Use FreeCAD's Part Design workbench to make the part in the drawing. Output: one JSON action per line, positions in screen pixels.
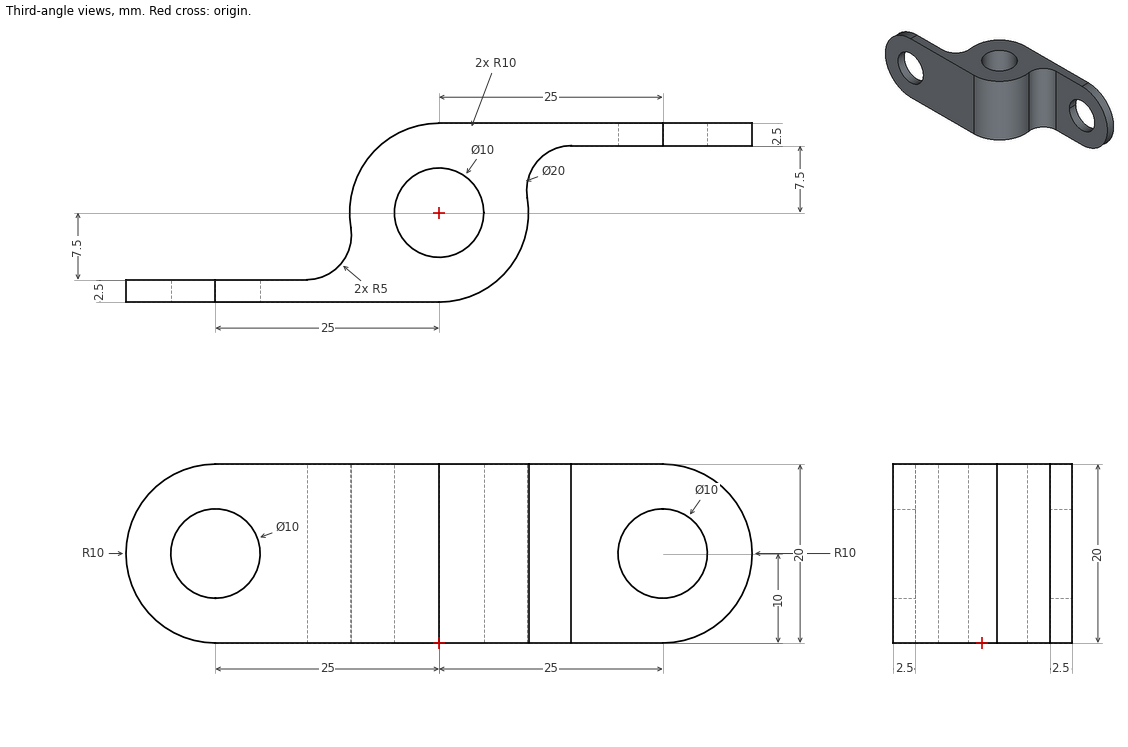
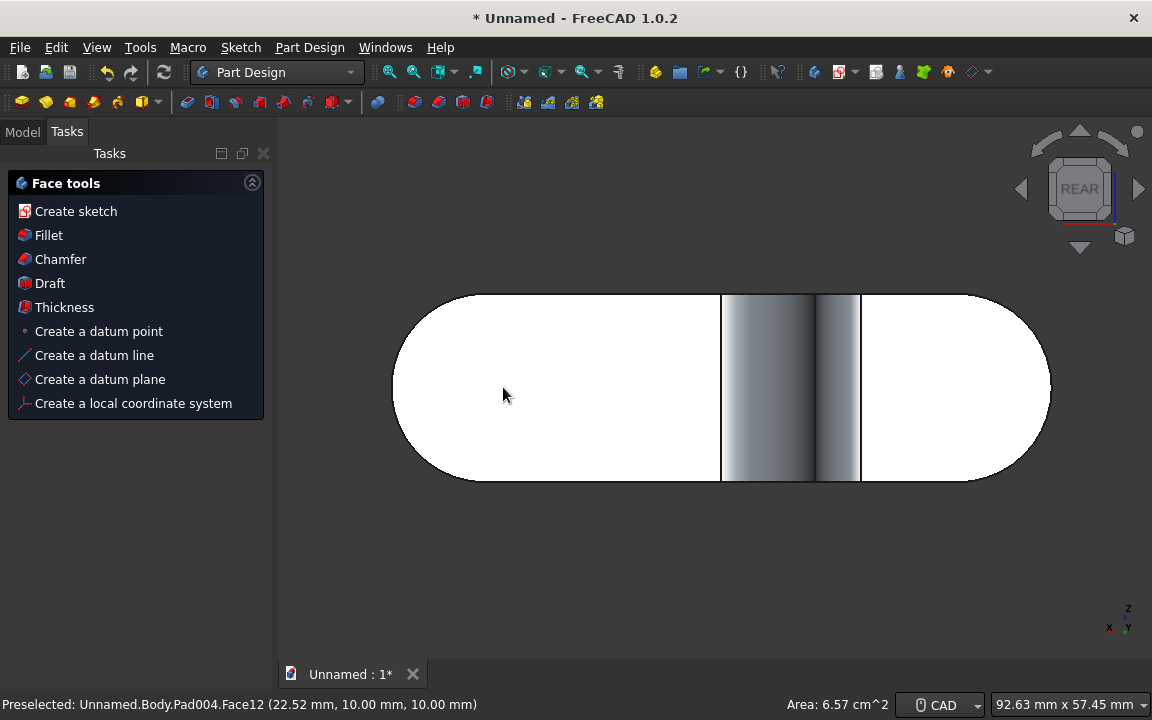
{"action": "left_click", "coordinate": [840, 72]}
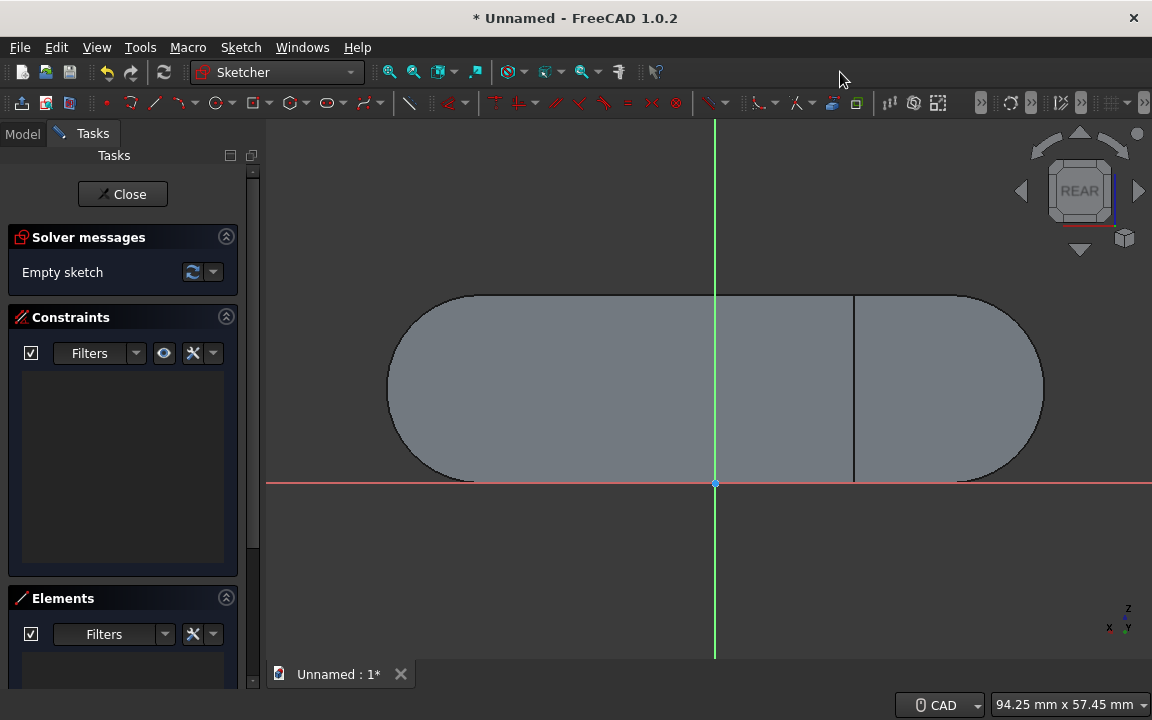
{"action": "scroll", "coordinate": [411, 389], "scroll_direction": "up", "scroll_amount": 6}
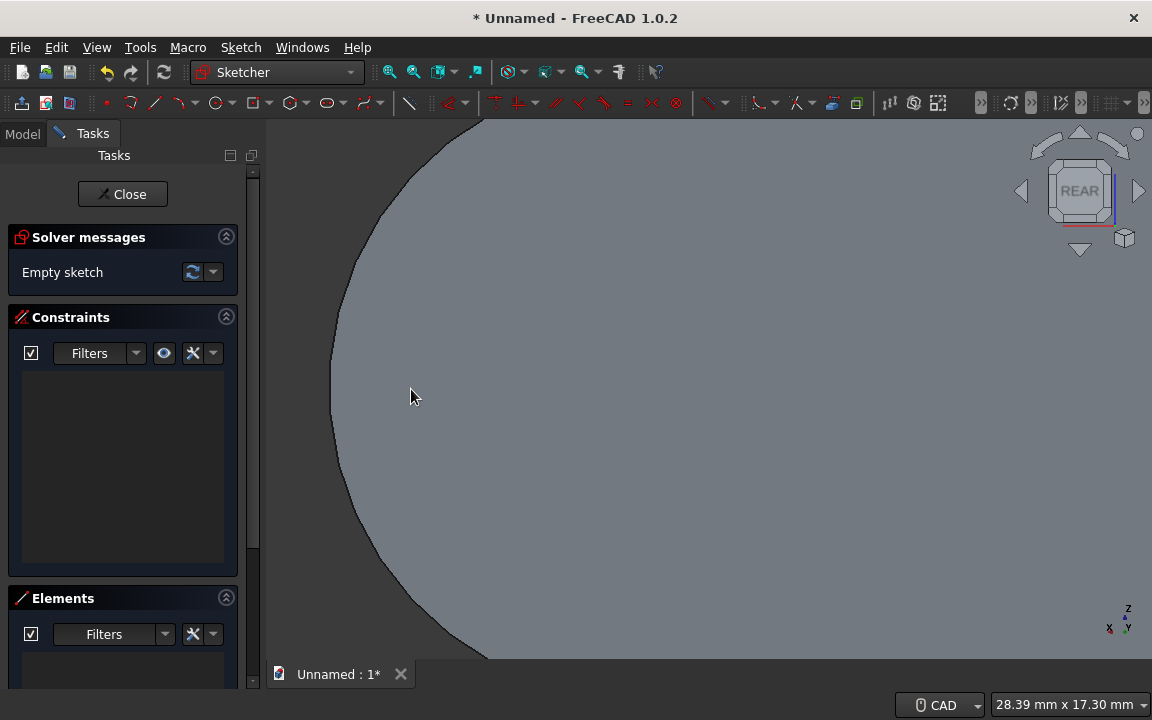
{"action": "key", "text": "g c"}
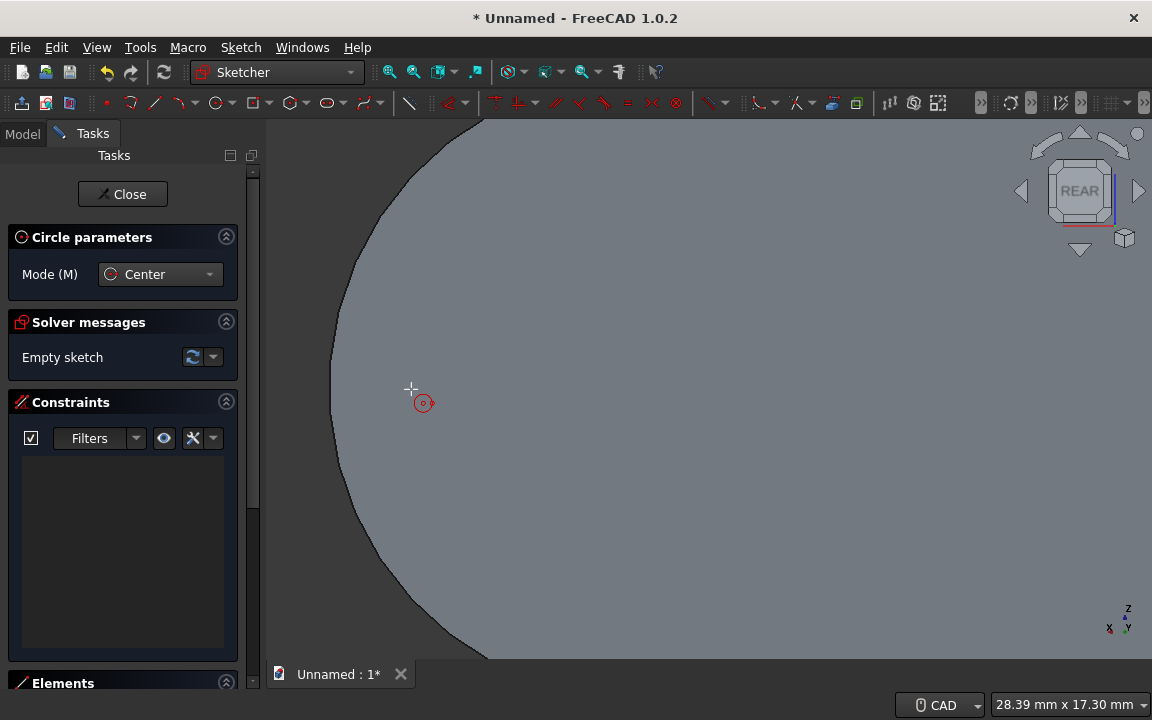
{"action": "left_click", "coordinate": [641, 388]}
{"action": "left_click", "coordinate": [752, 277]}
{"action": "key", "text": "Escape"}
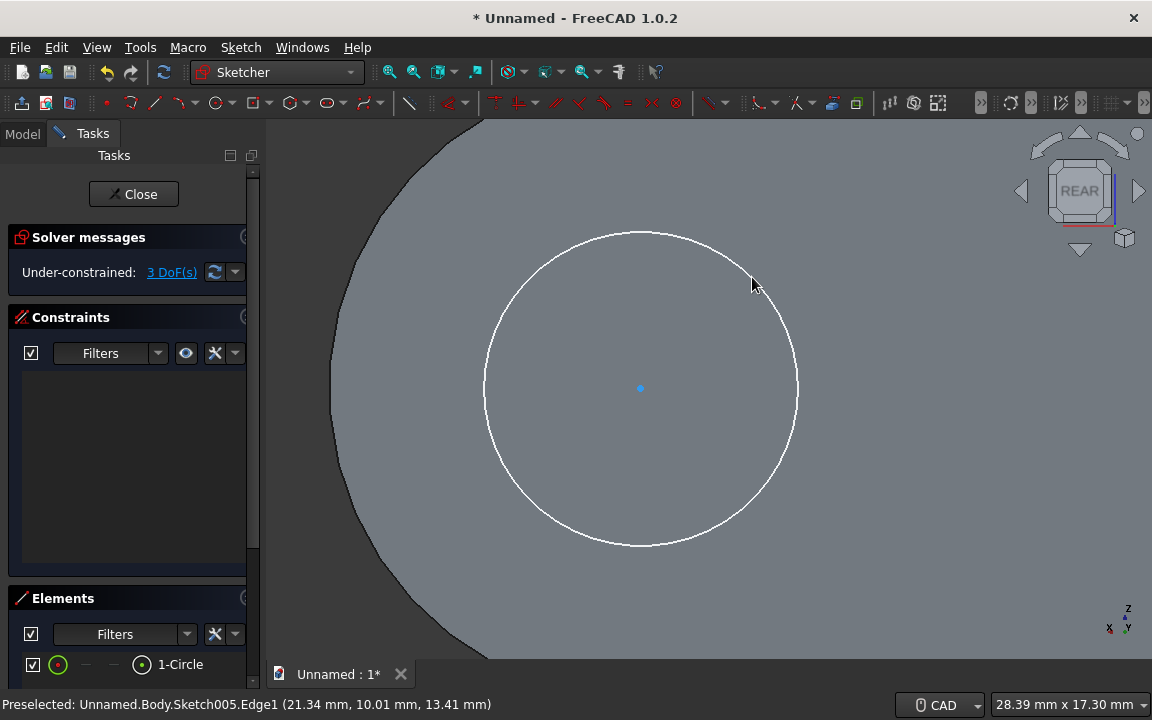
{"action": "key", "text": "d"}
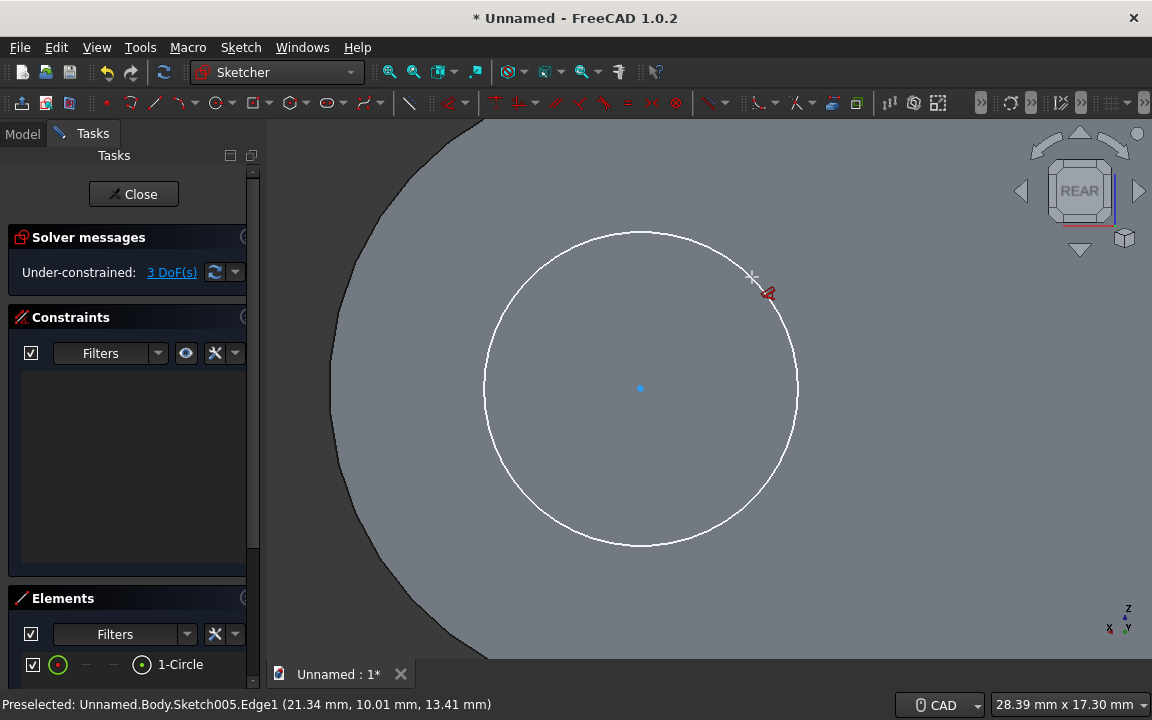
{"action": "left_click", "coordinate": [752, 278]}
{"action": "left_click", "coordinate": [775, 255]}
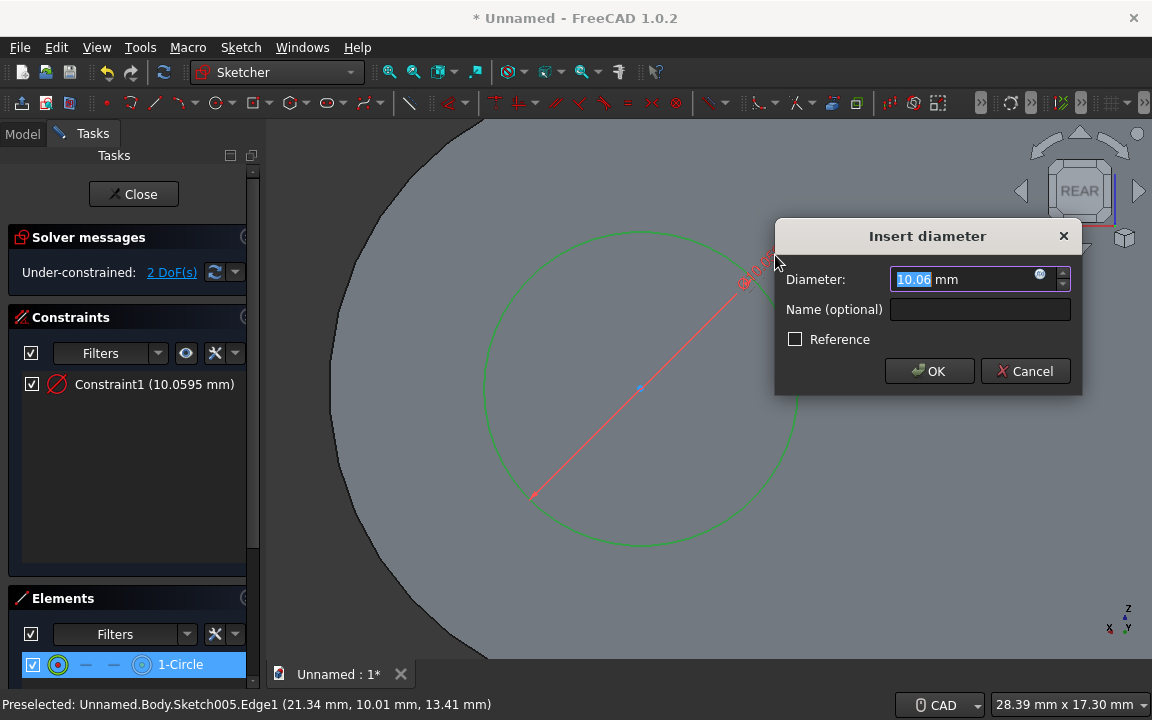
{"action": "type", "text": "10"}
{"action": "key", "text": "Return"}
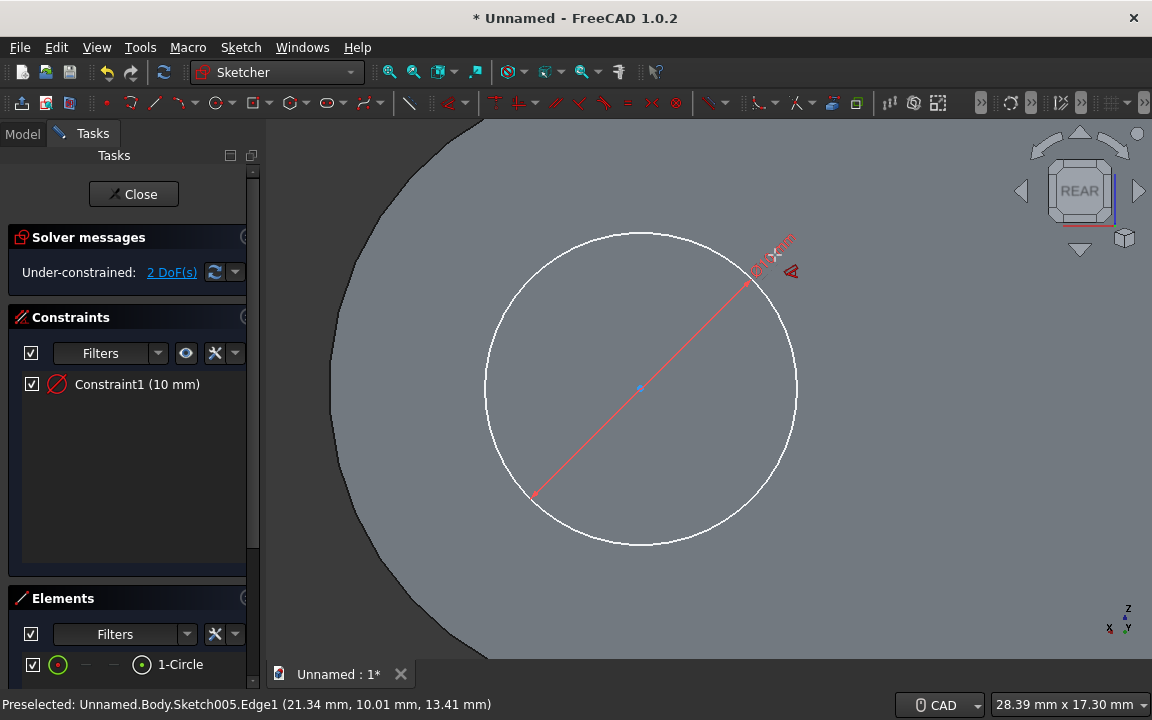
{"action": "left_click", "coordinate": [641, 389]}
{"action": "left_click", "coordinate": [814, 355]}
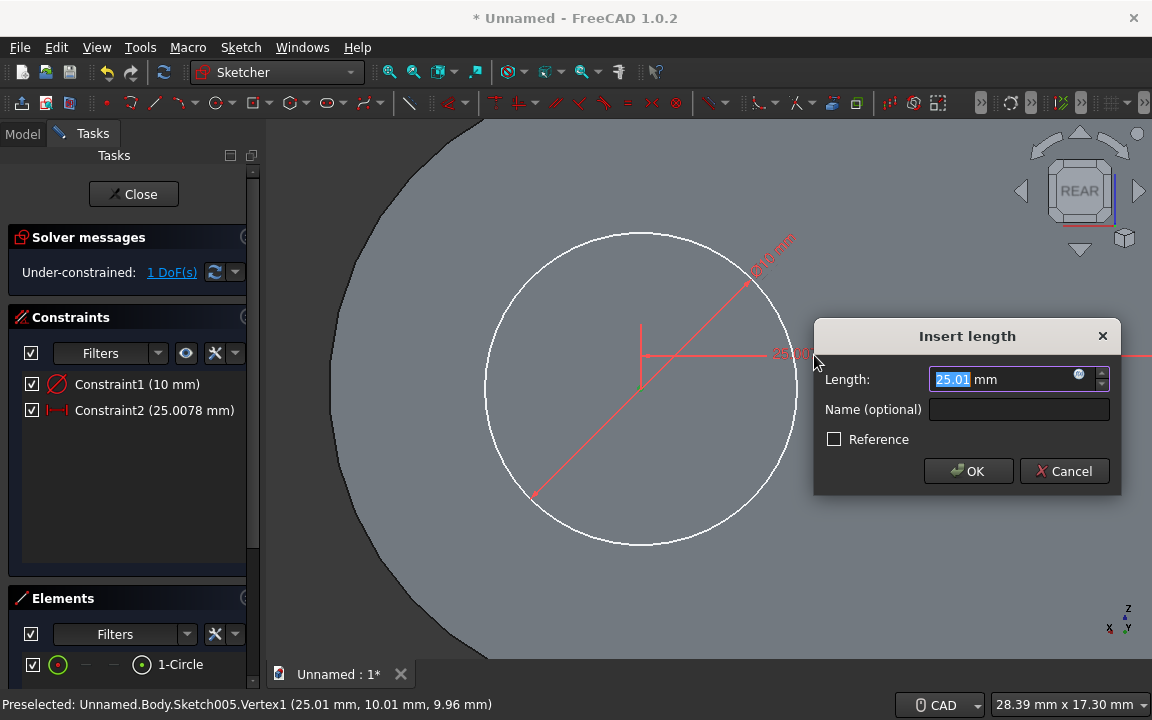
{"action": "type", "text": "25"}
{"action": "key", "text": "Return"}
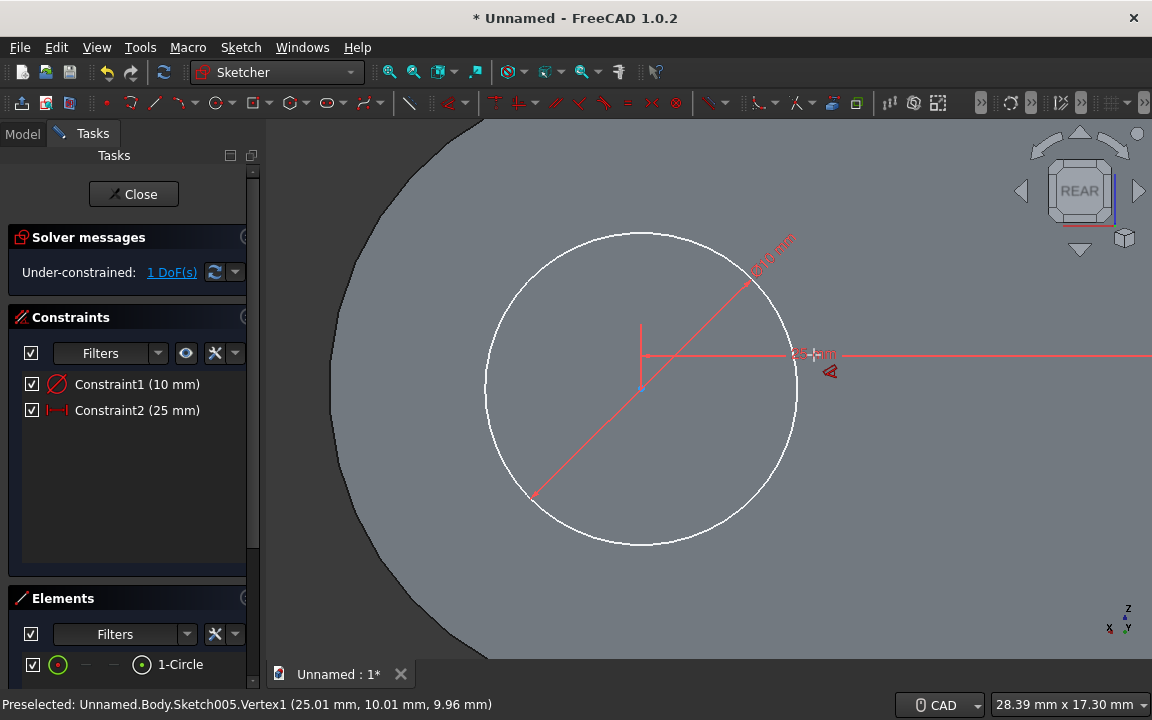
{"action": "left_click", "coordinate": [641, 389]}
{"action": "left_click", "coordinate": [607, 510]}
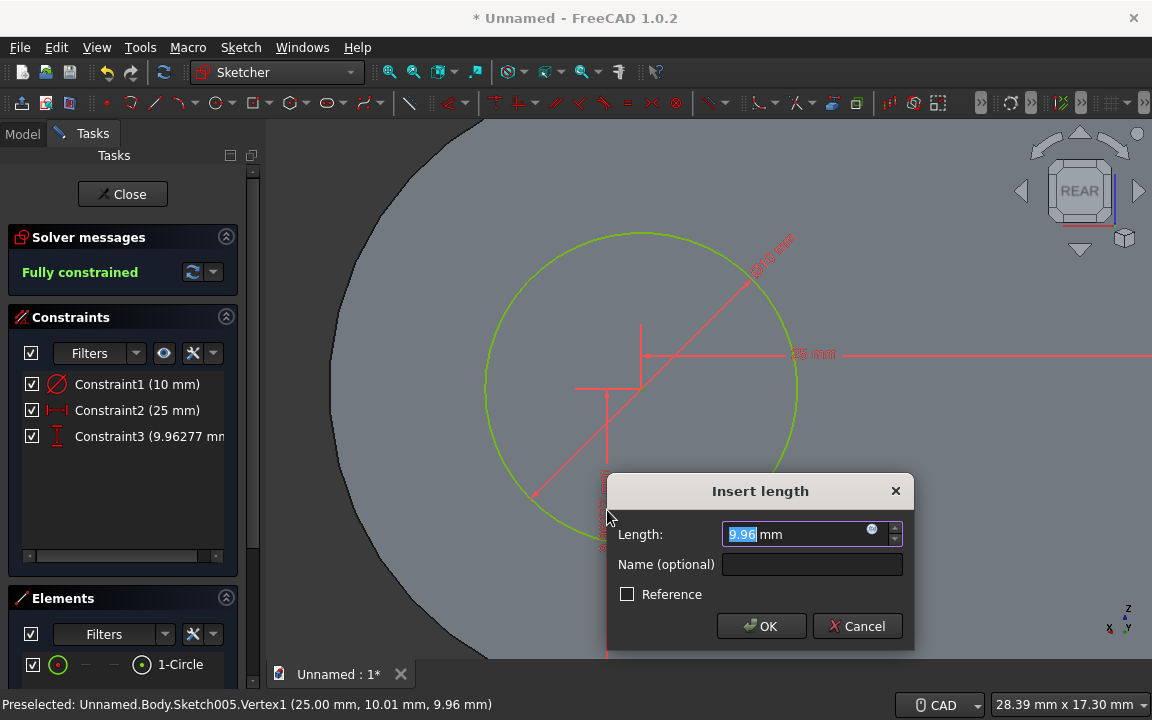
{"action": "type", "text": "10"}
{"action": "key", "text": "Return"}
{"action": "key", "text": "Escape"}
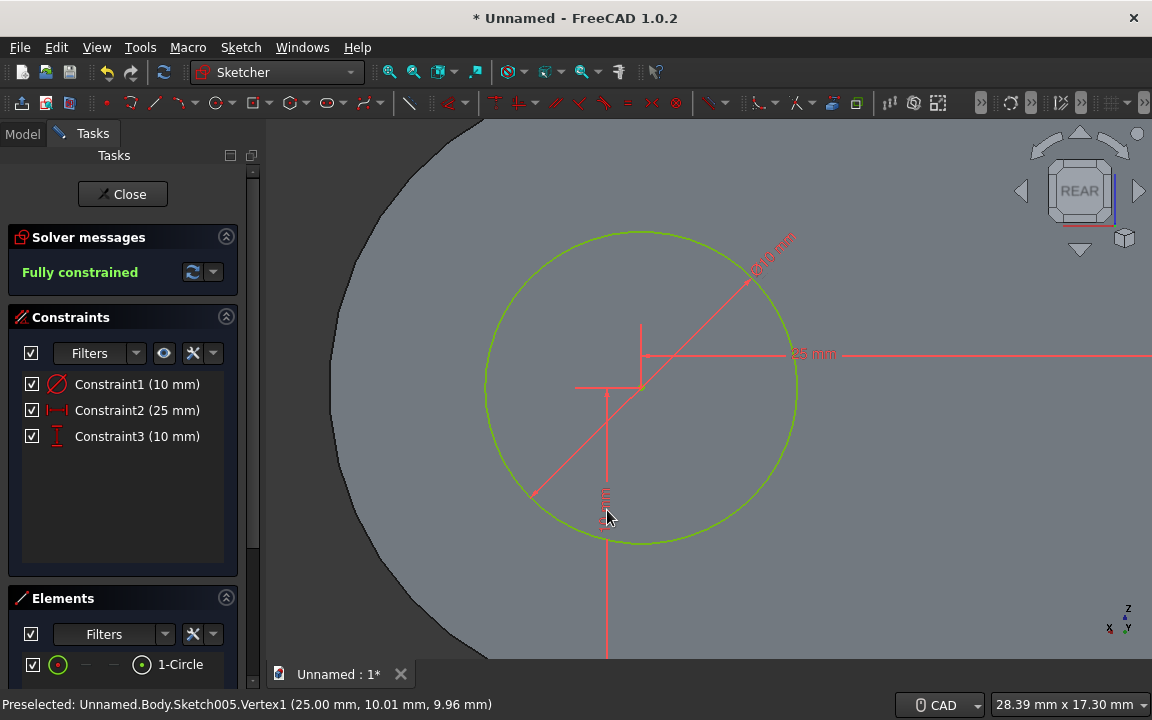
{"action": "left_click", "coordinate": [123, 194]}